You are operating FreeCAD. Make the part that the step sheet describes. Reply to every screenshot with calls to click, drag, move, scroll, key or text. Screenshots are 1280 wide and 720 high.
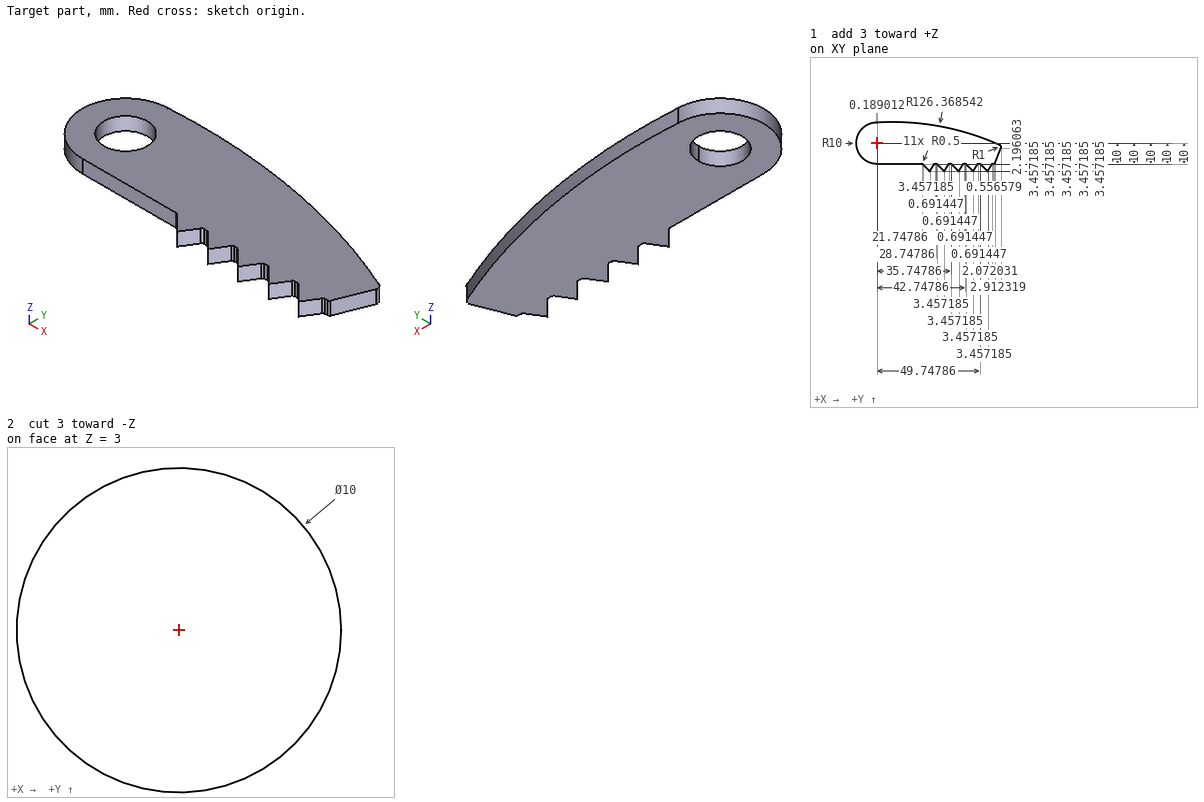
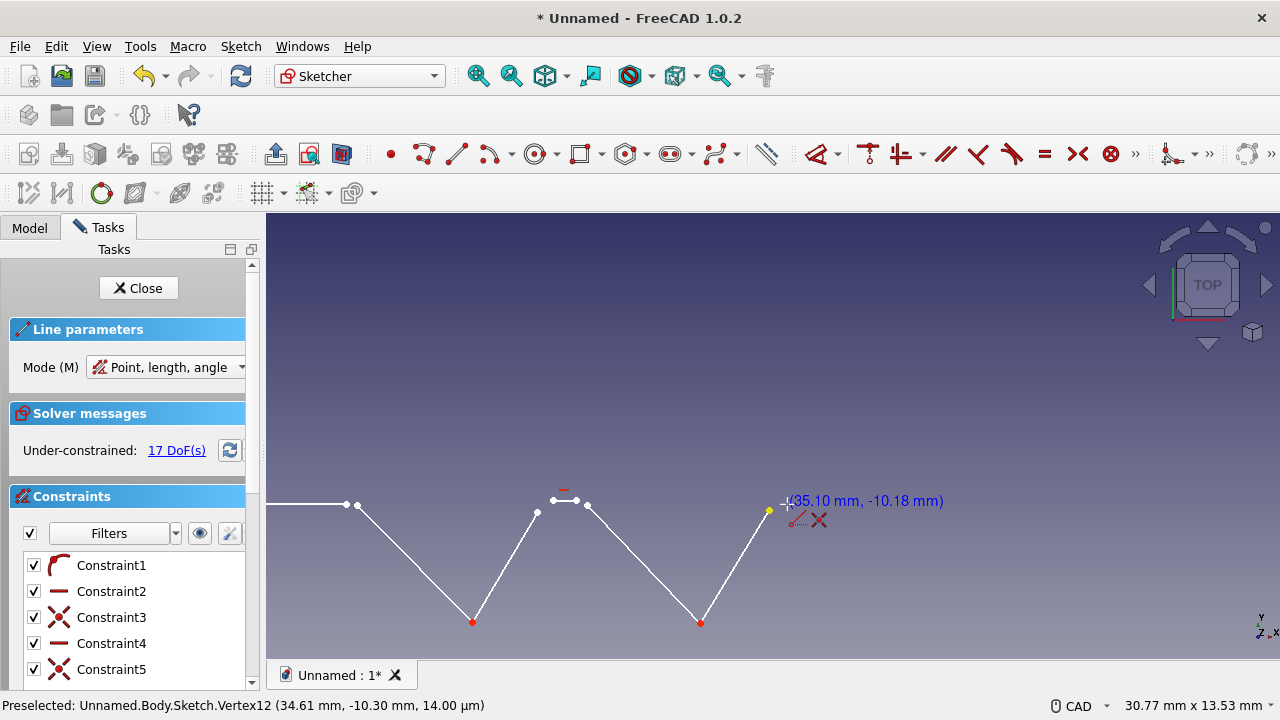
click(784, 500)
click(807, 500)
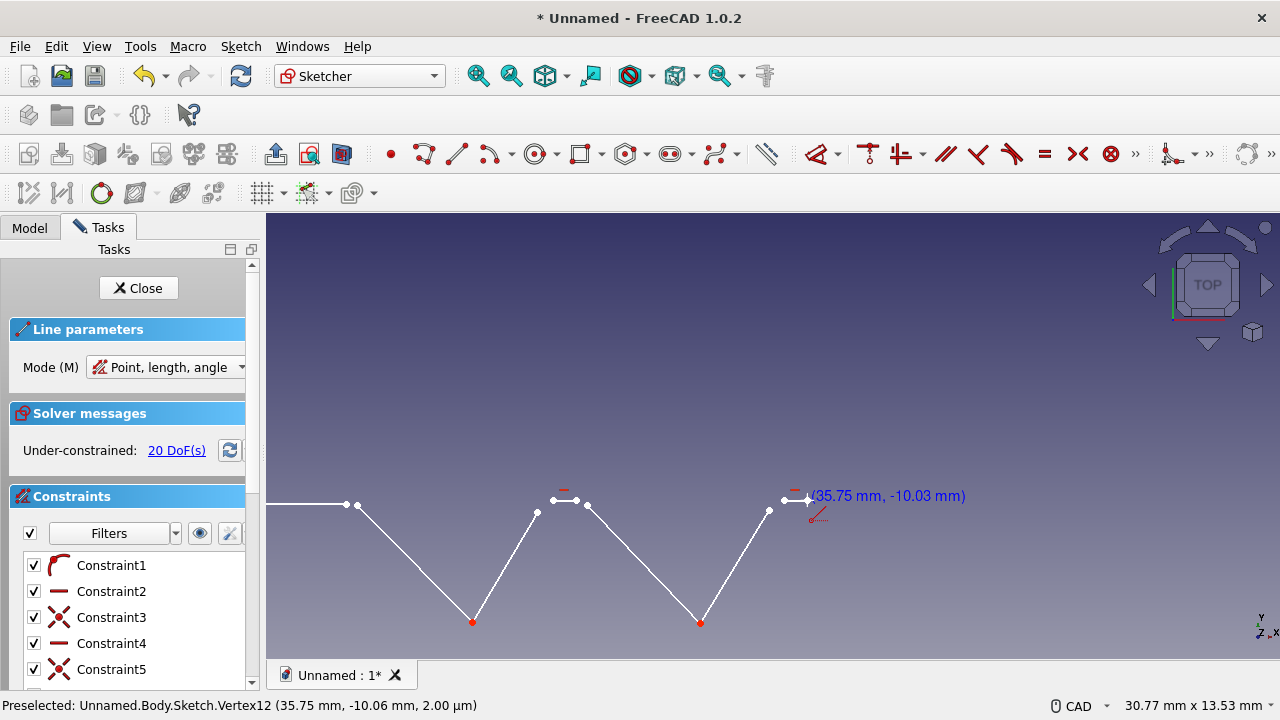
key(g)
key(m)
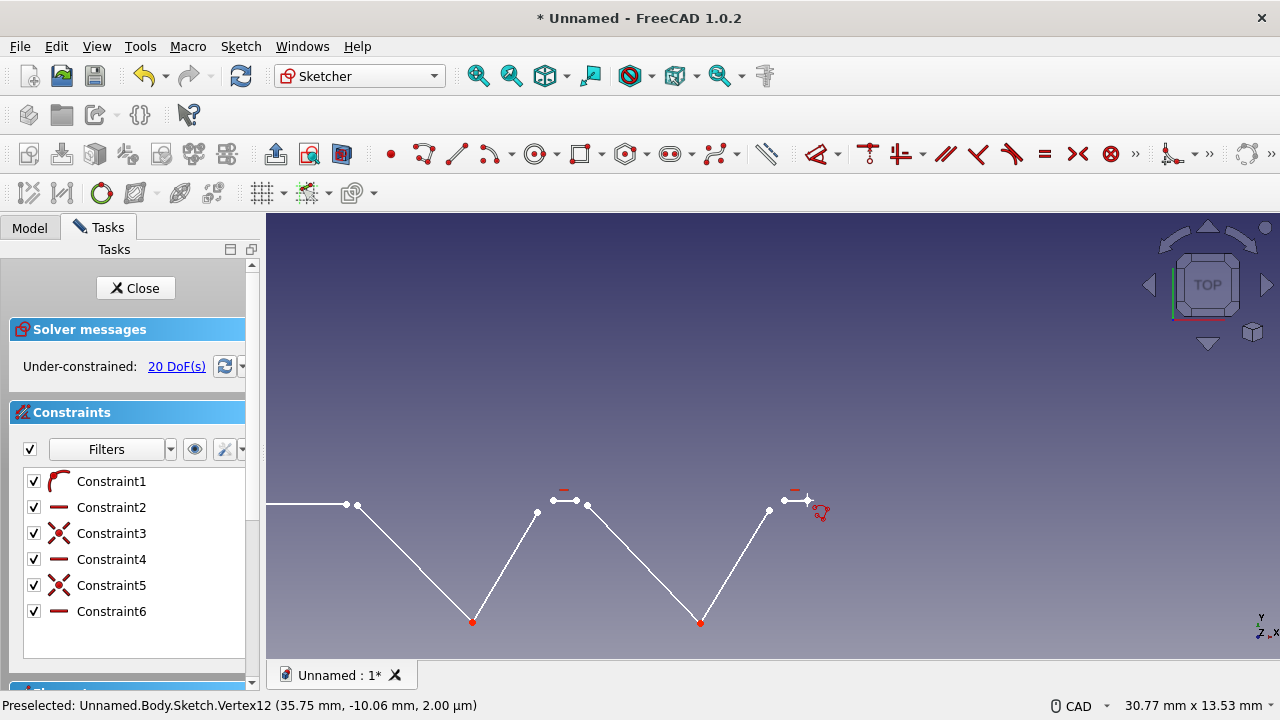
scroll(818, 505, up, 2)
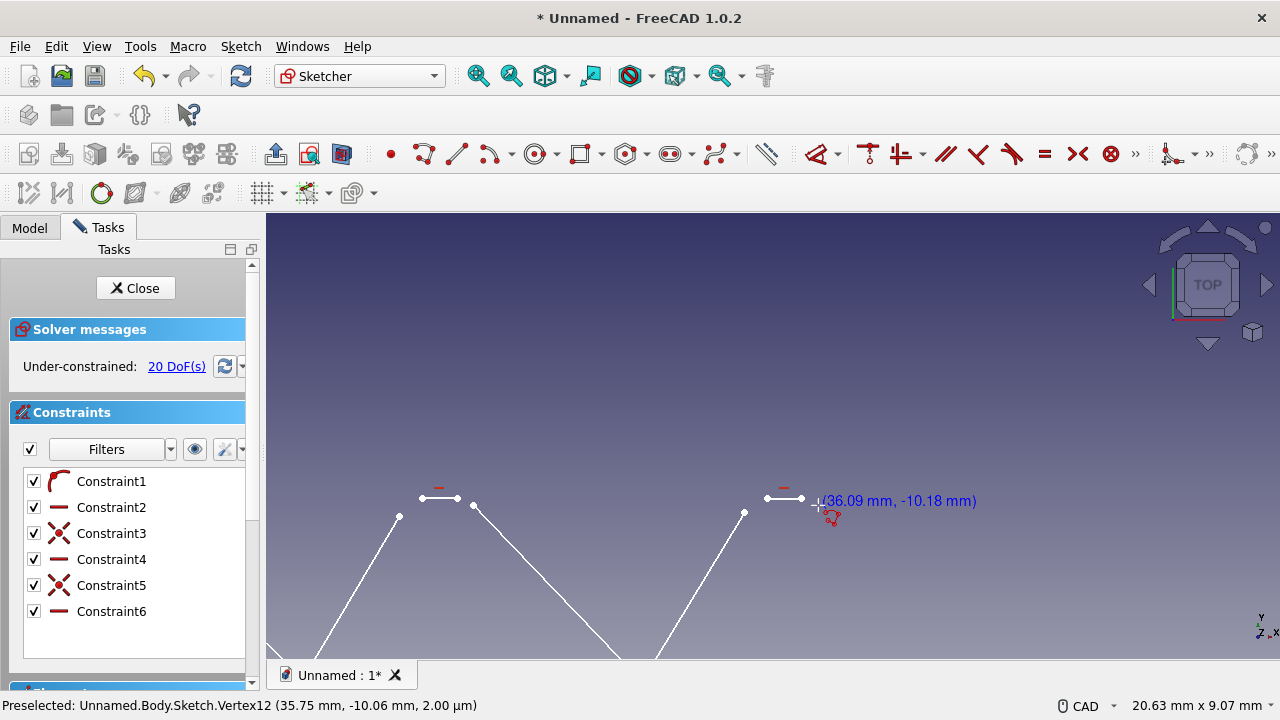
click(818, 505)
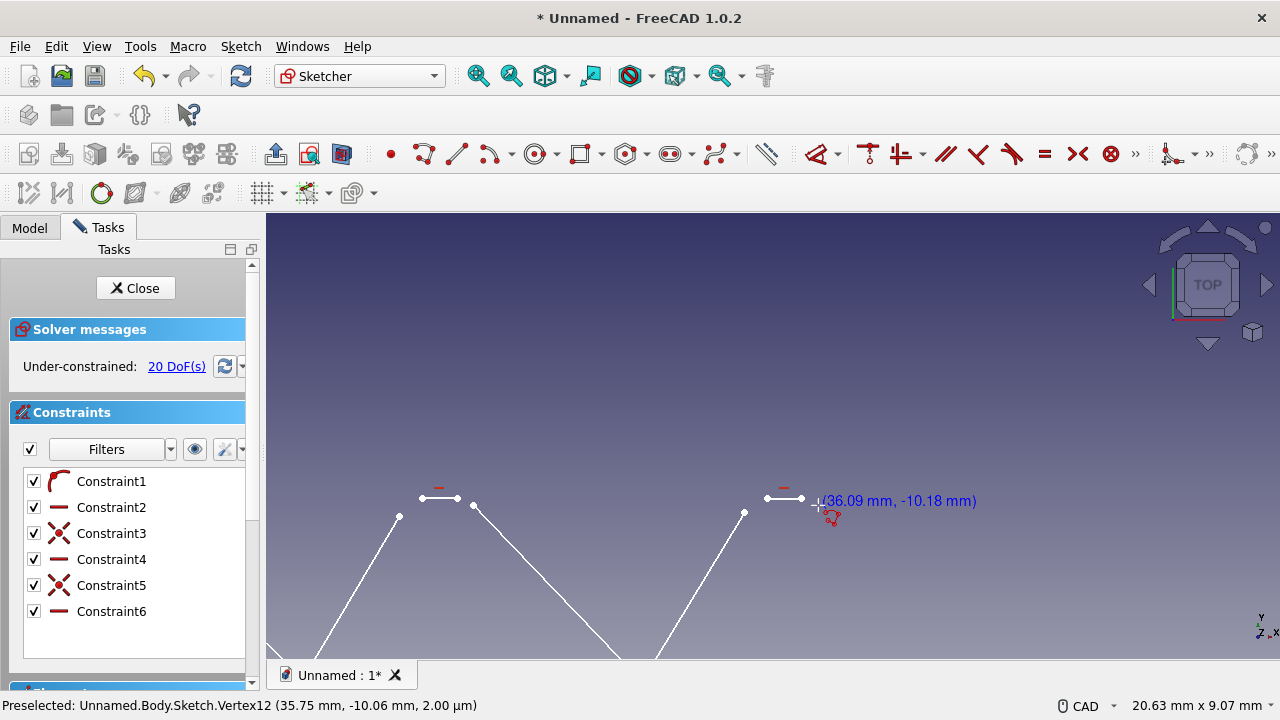
scroll(790, 504, down, 9)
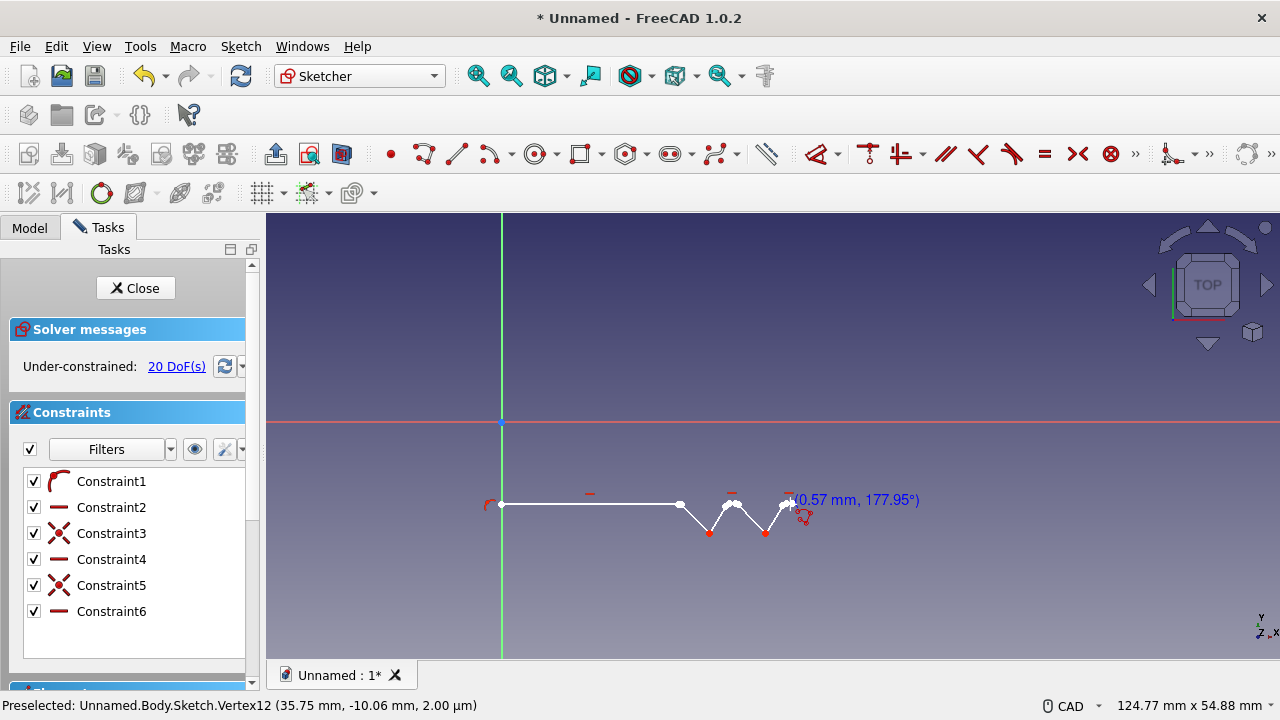
click(823, 533)
click(840, 505)
right_click(840, 505)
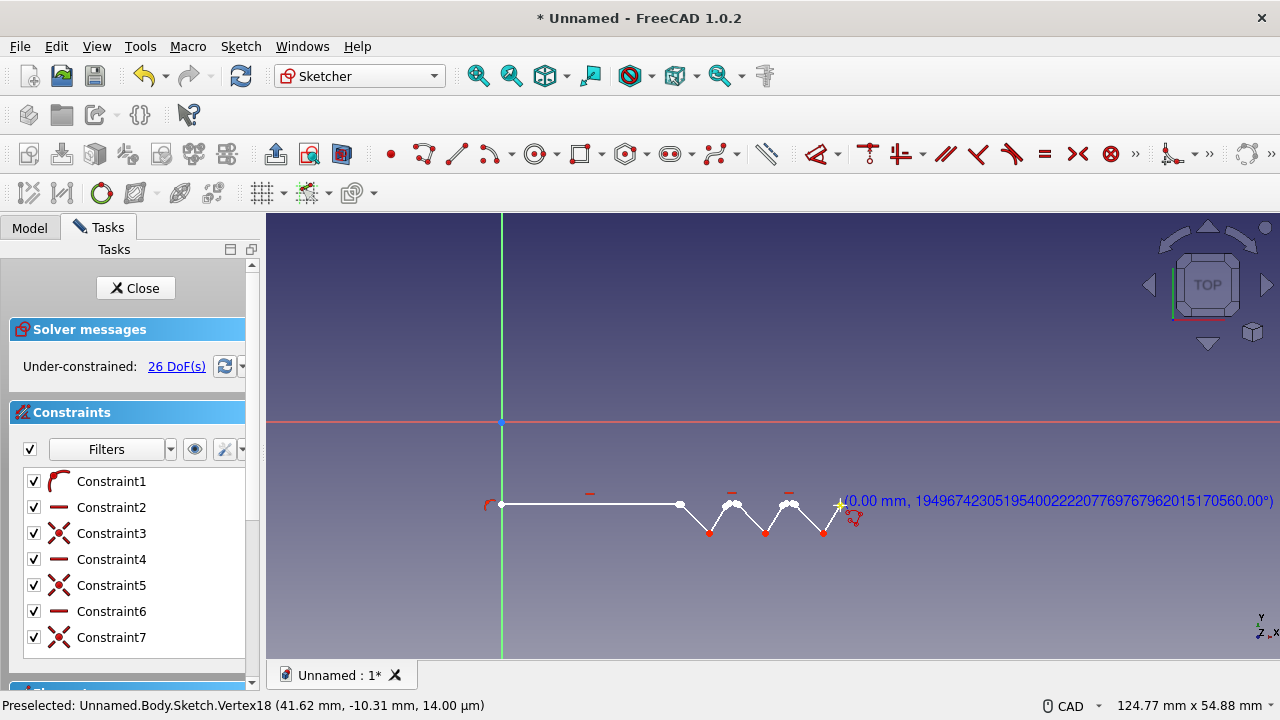
click(457, 154)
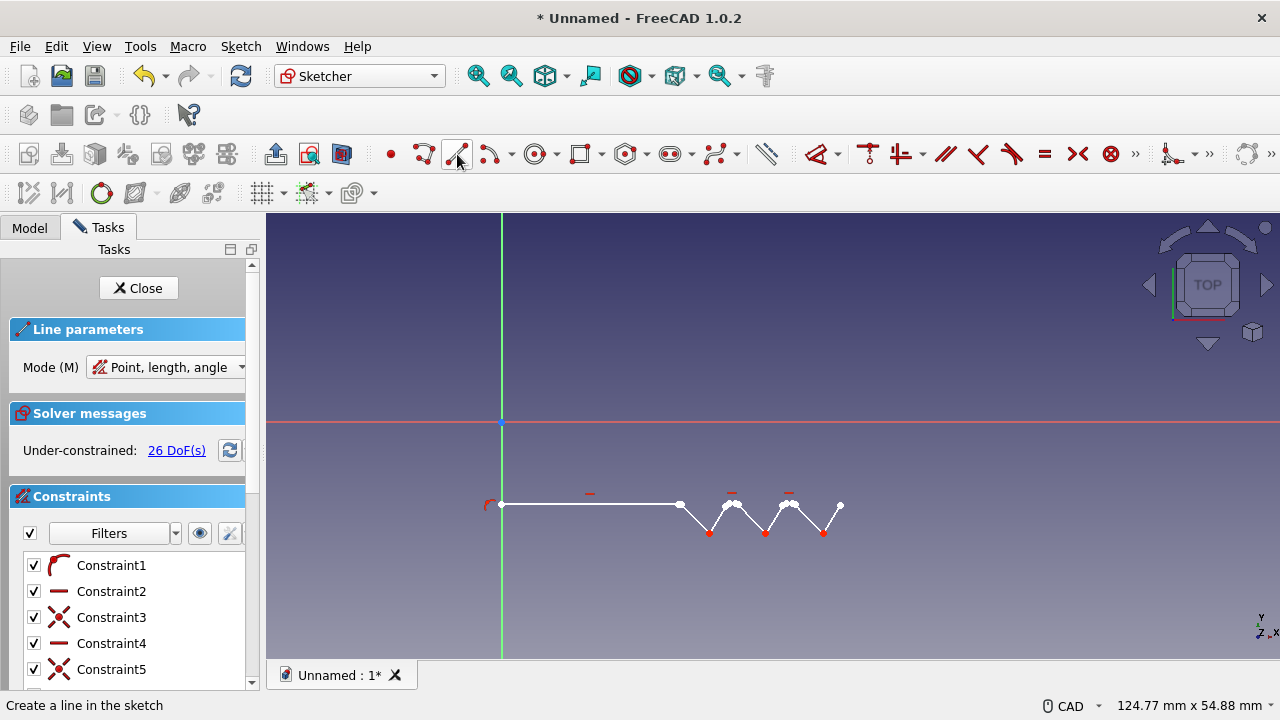
scroll(844, 503, up, 7)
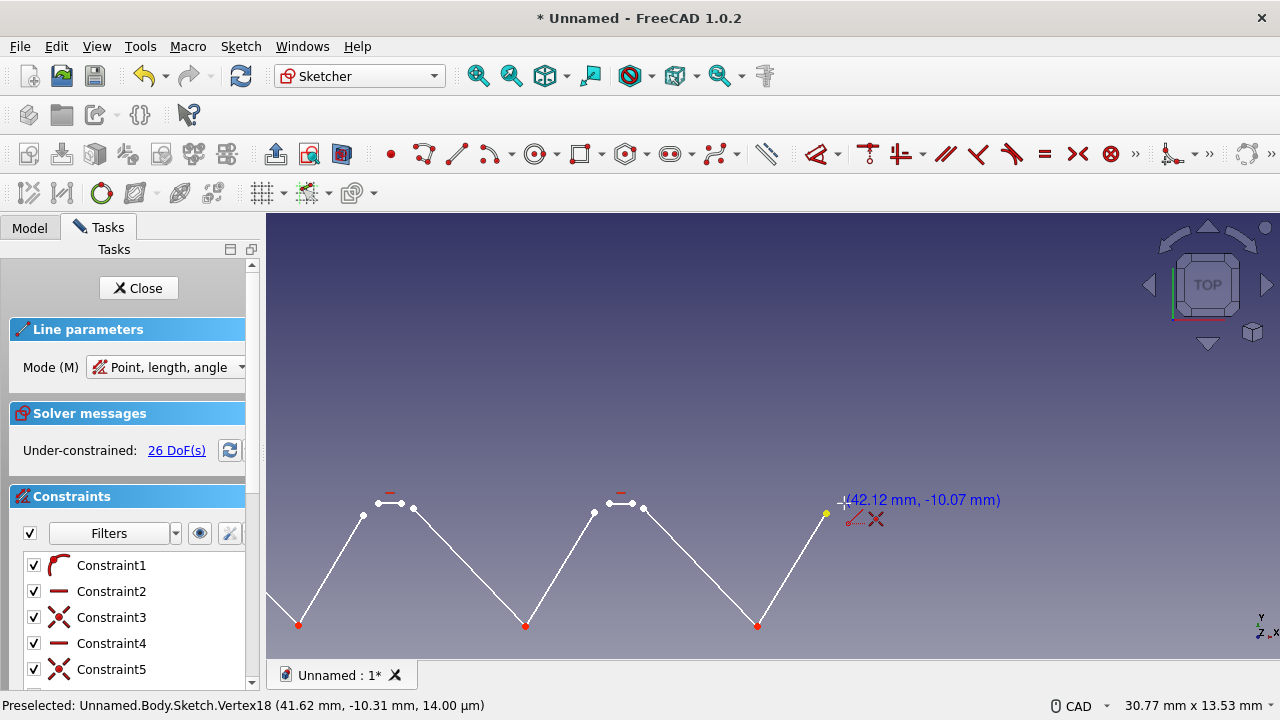
click(840, 503)
click(863, 503)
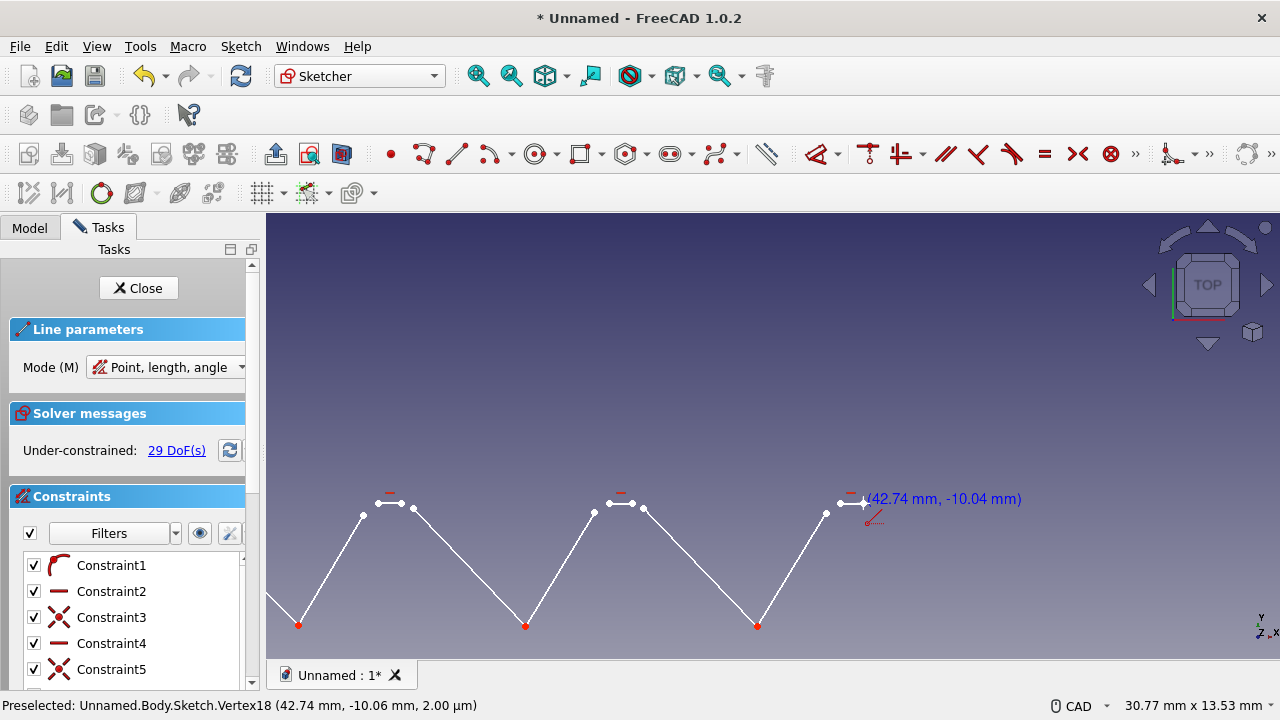
click(424, 154)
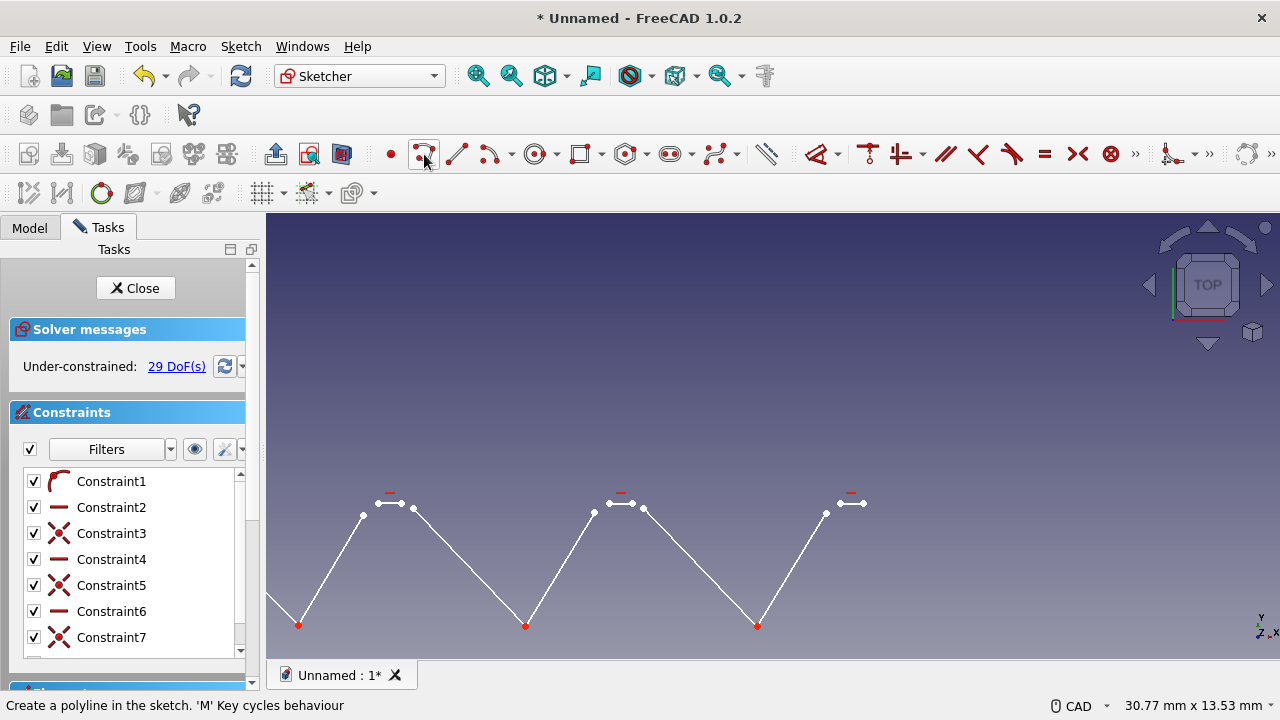
scroll(875, 508, up, 2)